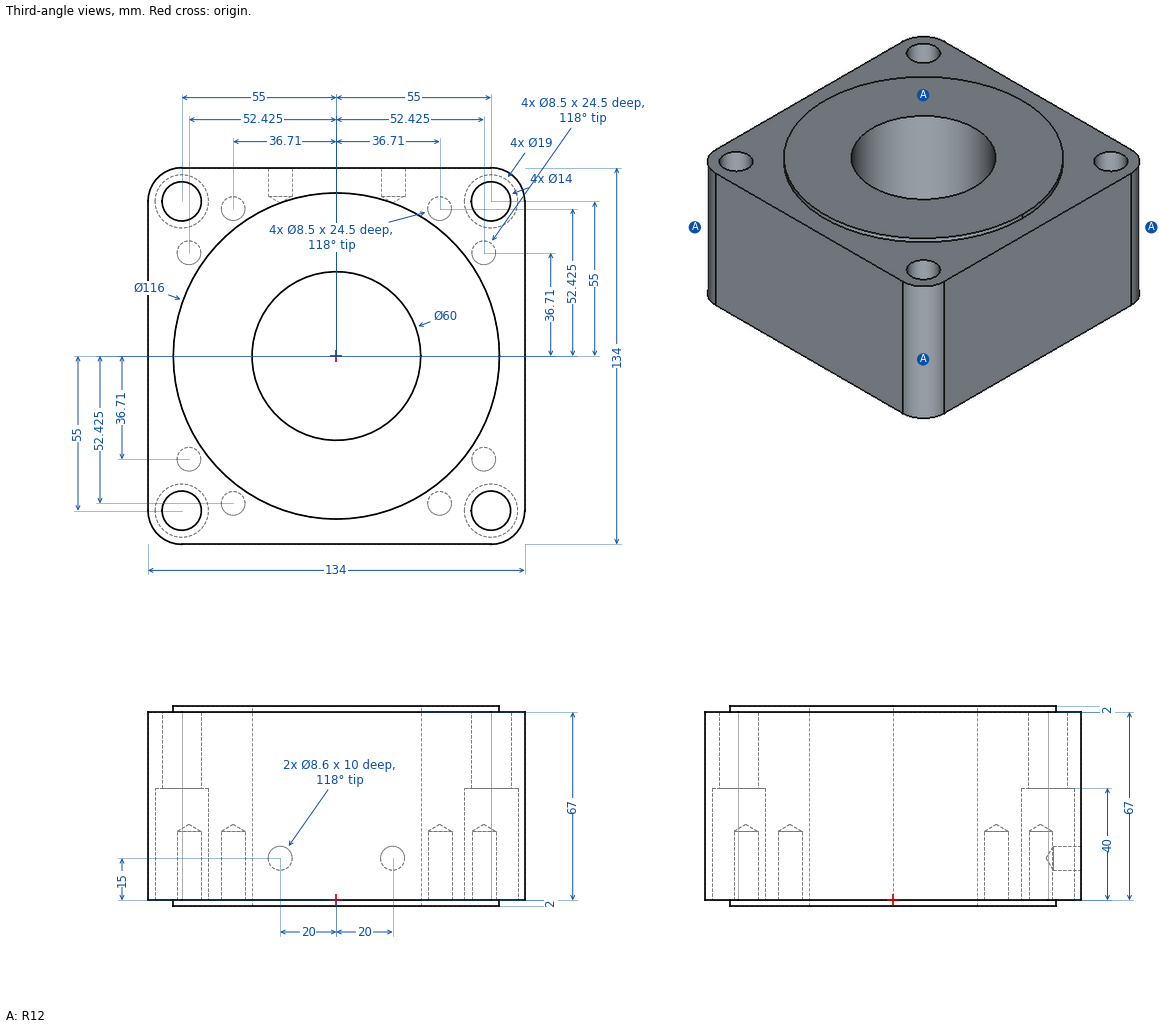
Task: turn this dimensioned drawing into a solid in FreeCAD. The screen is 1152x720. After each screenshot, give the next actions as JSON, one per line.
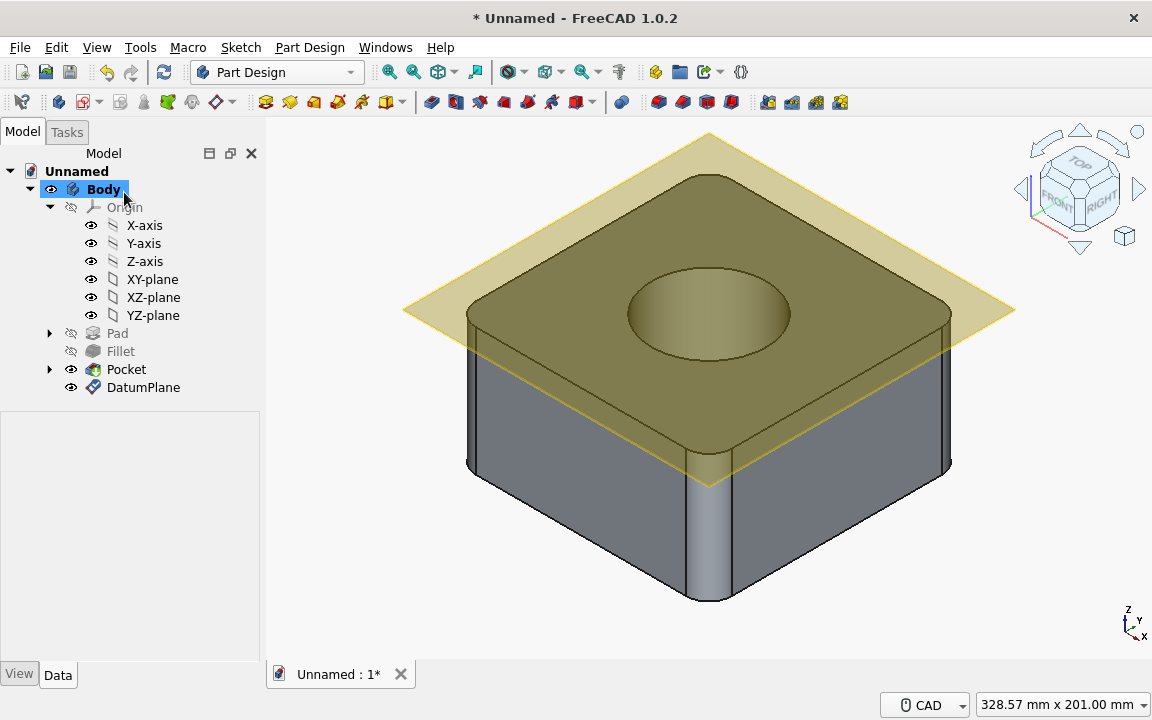
{"action": "left_click", "coordinate": [116, 387]}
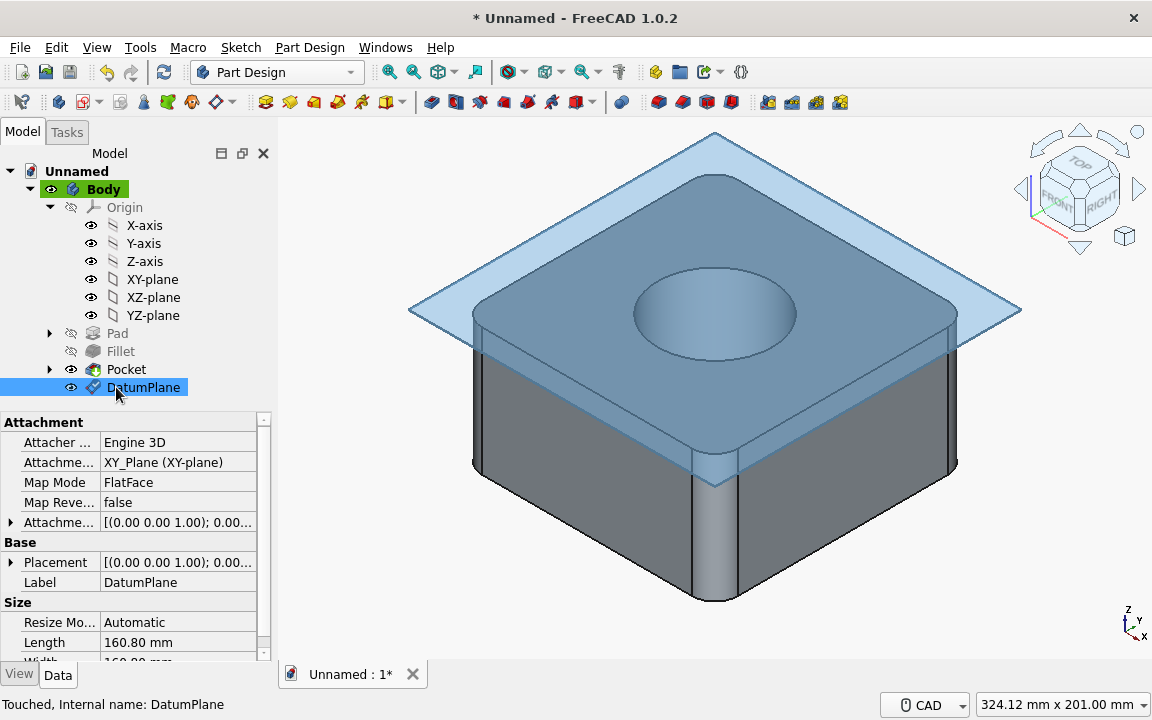
{"action": "left_click", "coordinate": [84, 102]}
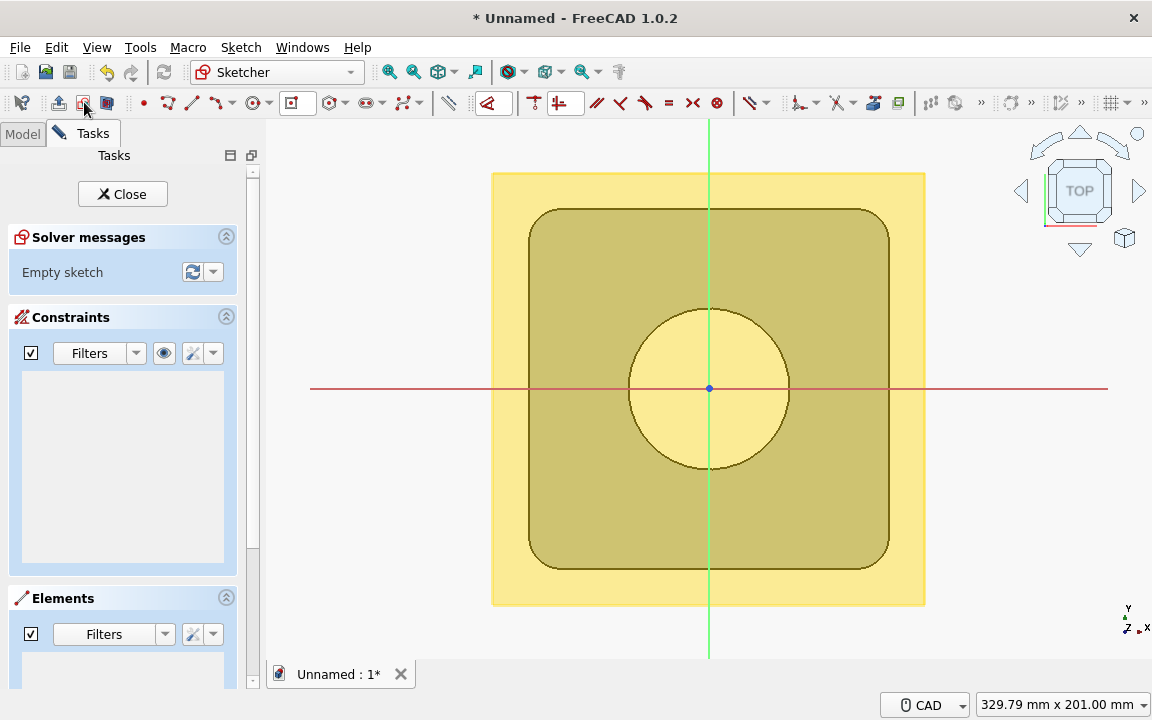
{"action": "left_click", "coordinate": [254, 104]}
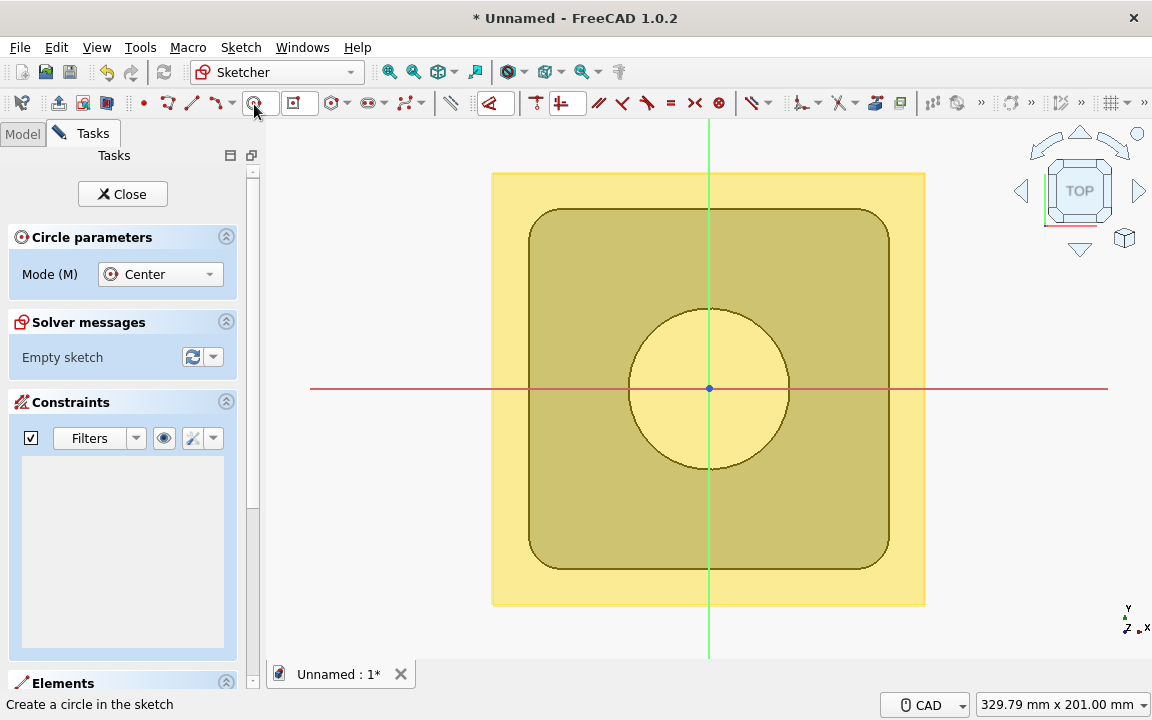
{"action": "left_click", "coordinate": [709, 389]}
{"action": "left_click", "coordinate": [819, 279]}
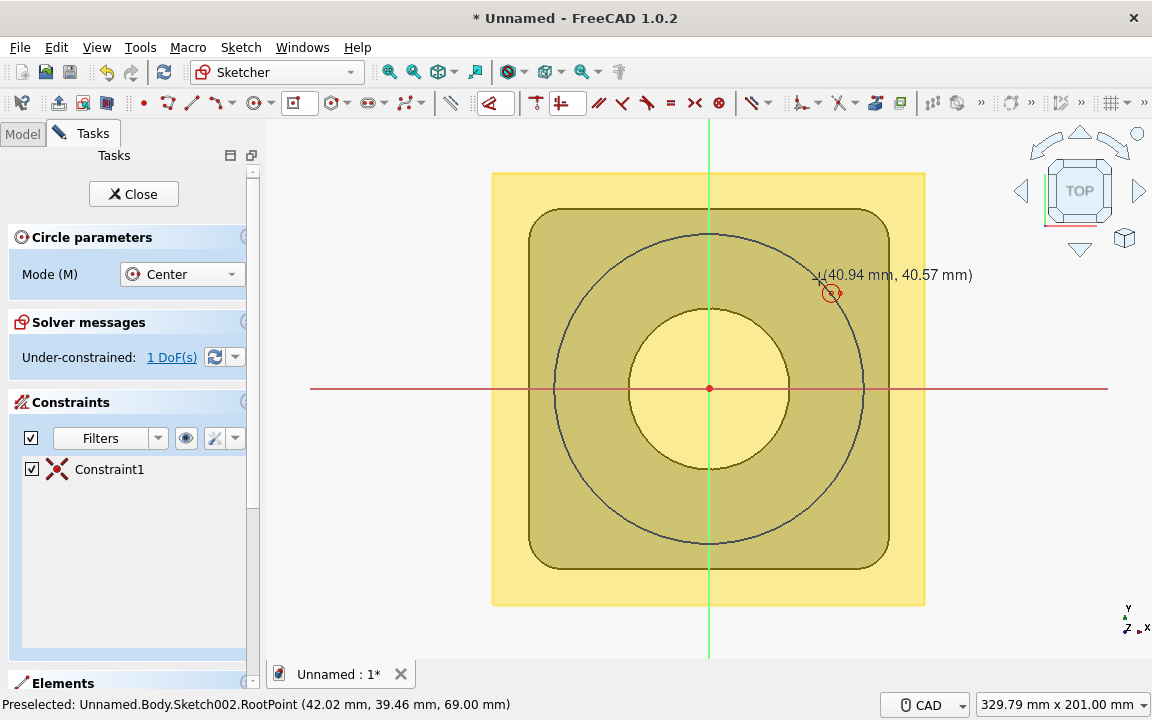
{"action": "left_click", "coordinate": [709, 389]}
{"action": "left_click", "coordinate": [766, 332]}
{"action": "key", "text": "Escape"}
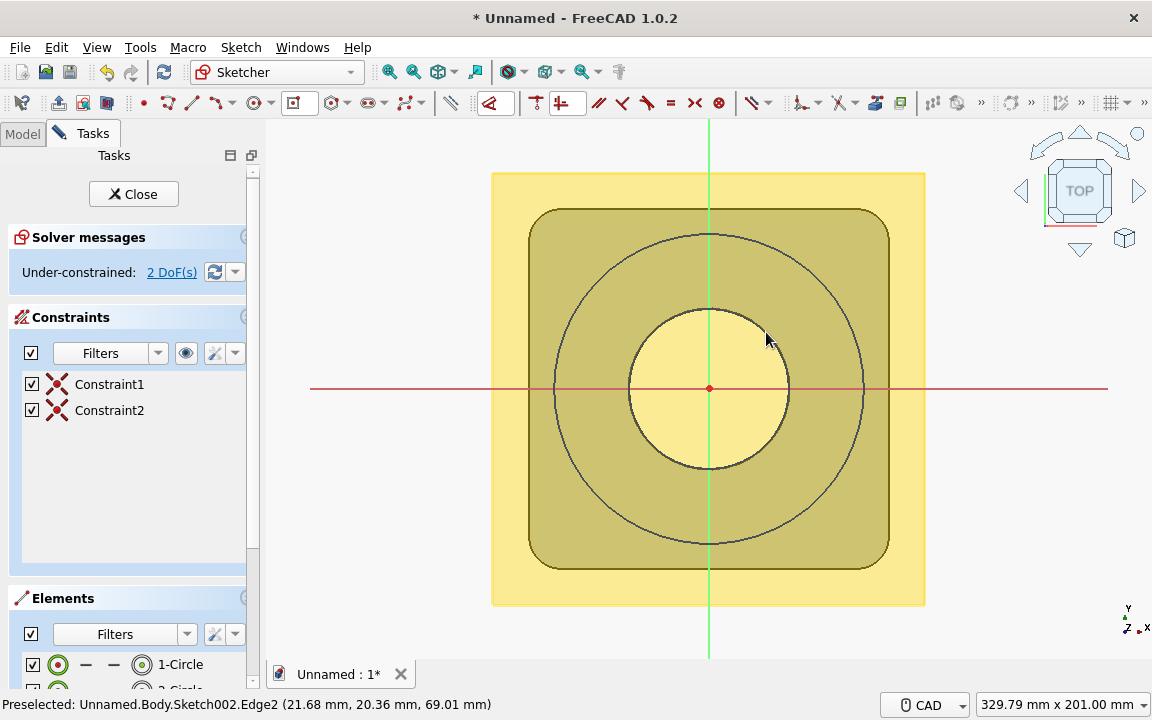
{"action": "left_click", "coordinate": [818, 279]}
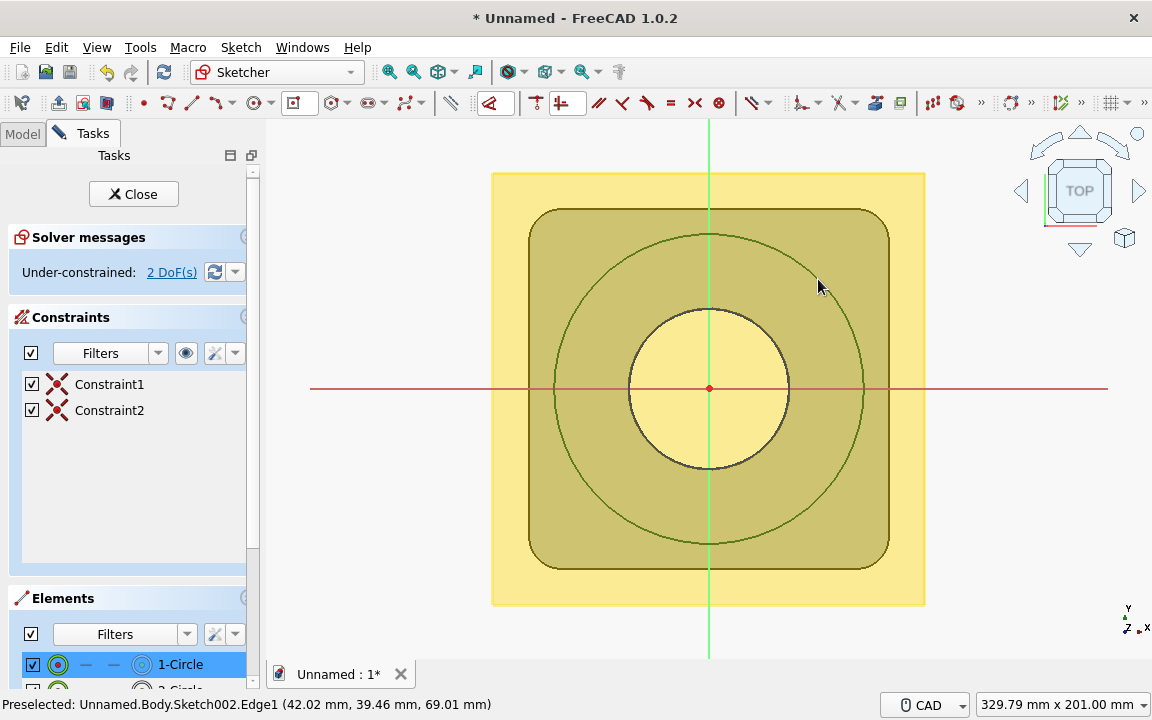
{"action": "left_click", "coordinate": [508, 104]}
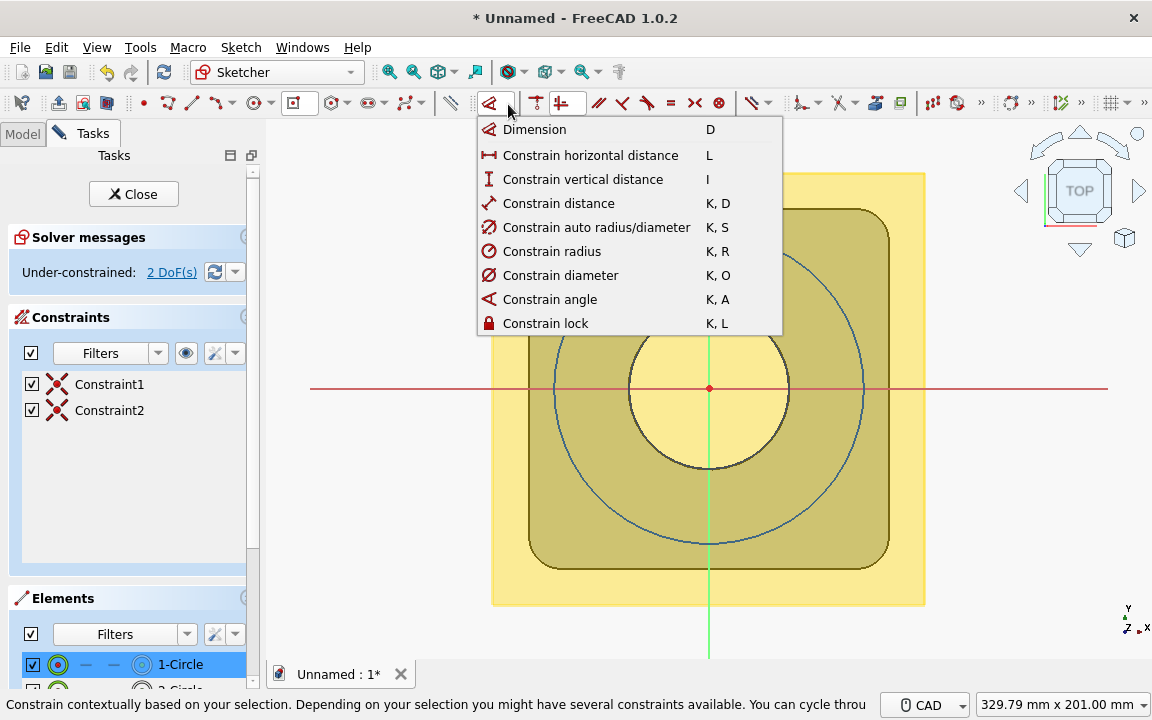
{"action": "left_click", "coordinate": [630, 275]}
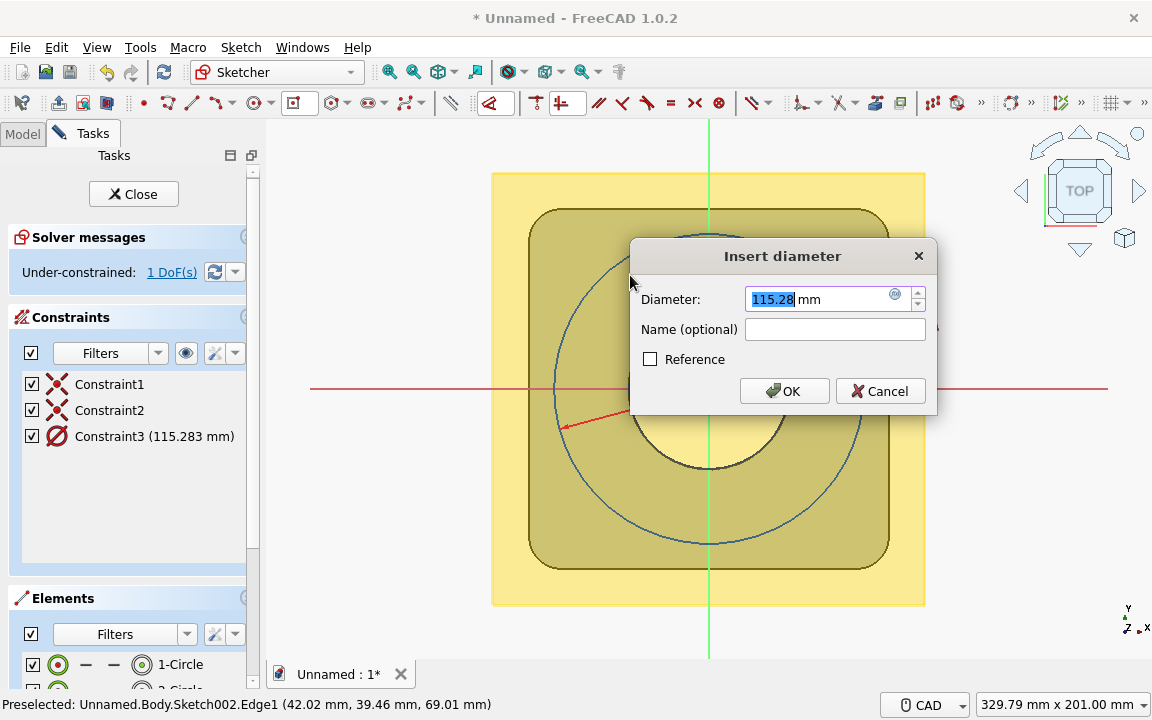
{"action": "type", "text": "116"}
{"action": "key", "text": "Return"}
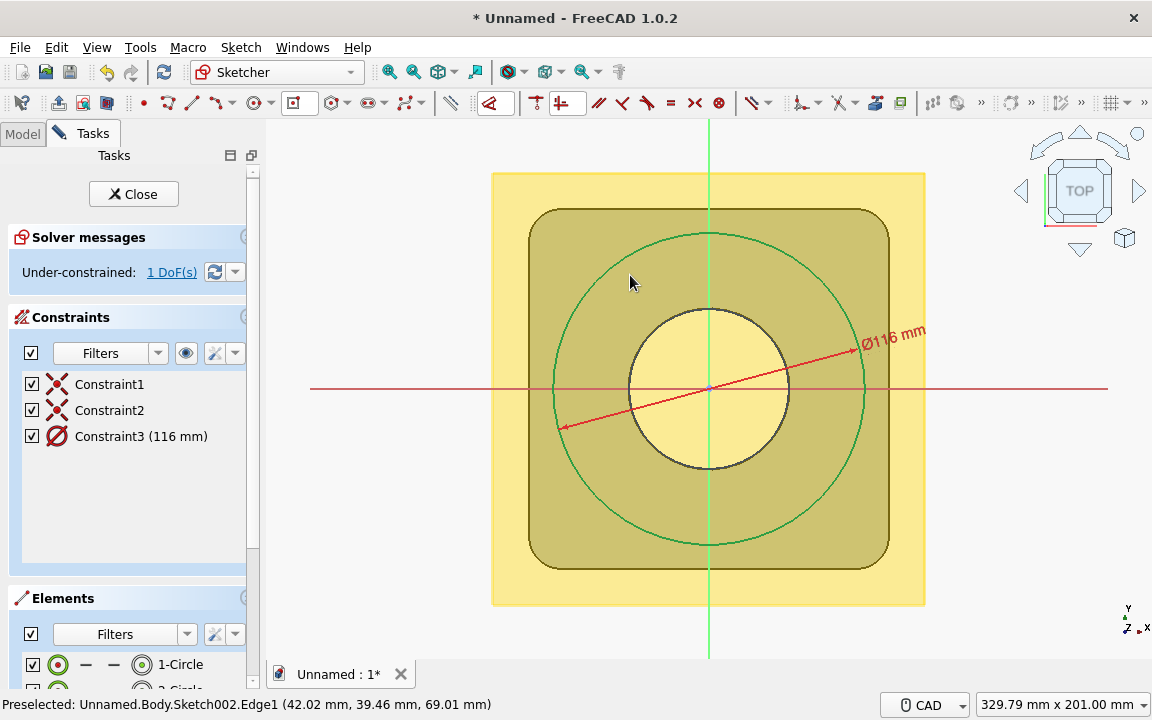
{"action": "left_click", "coordinate": [765, 332]}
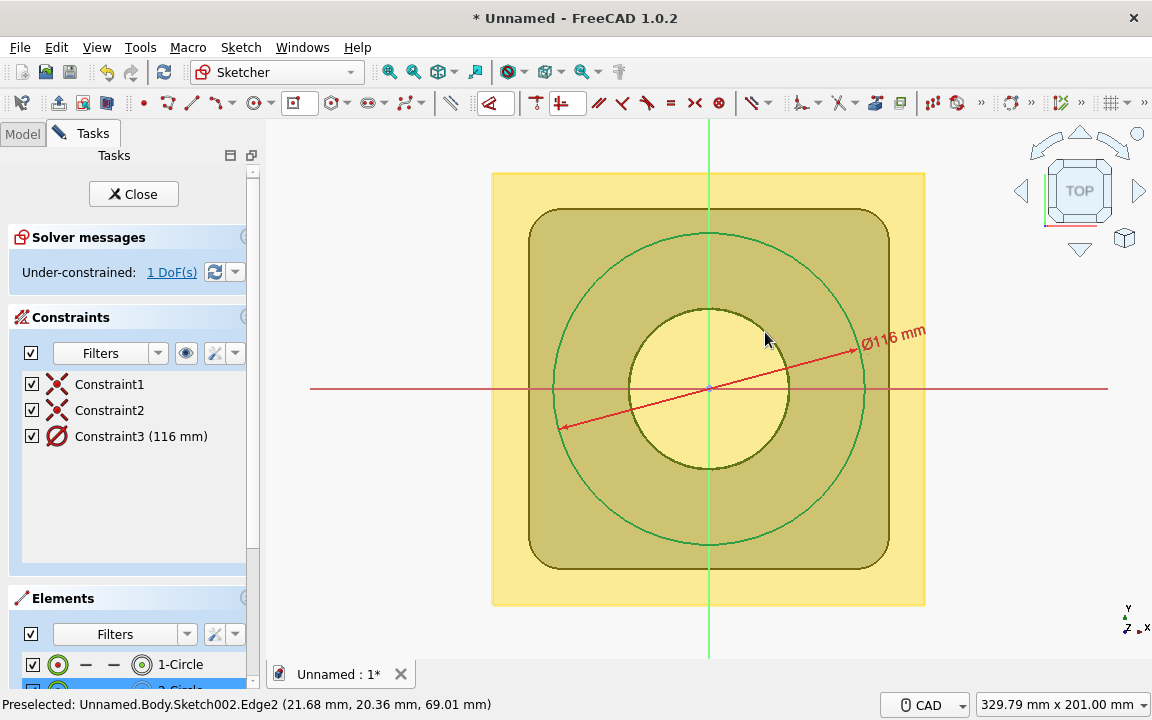
{"action": "left_click", "coordinate": [508, 104]}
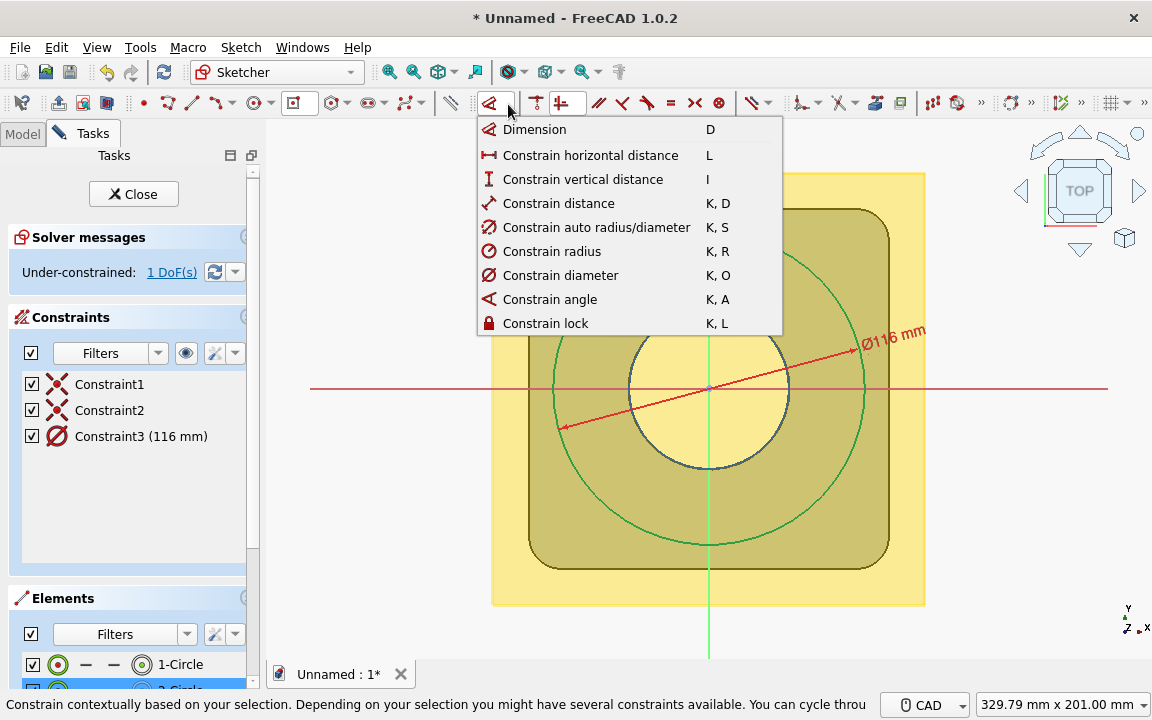
{"action": "left_click", "coordinate": [630, 275]}